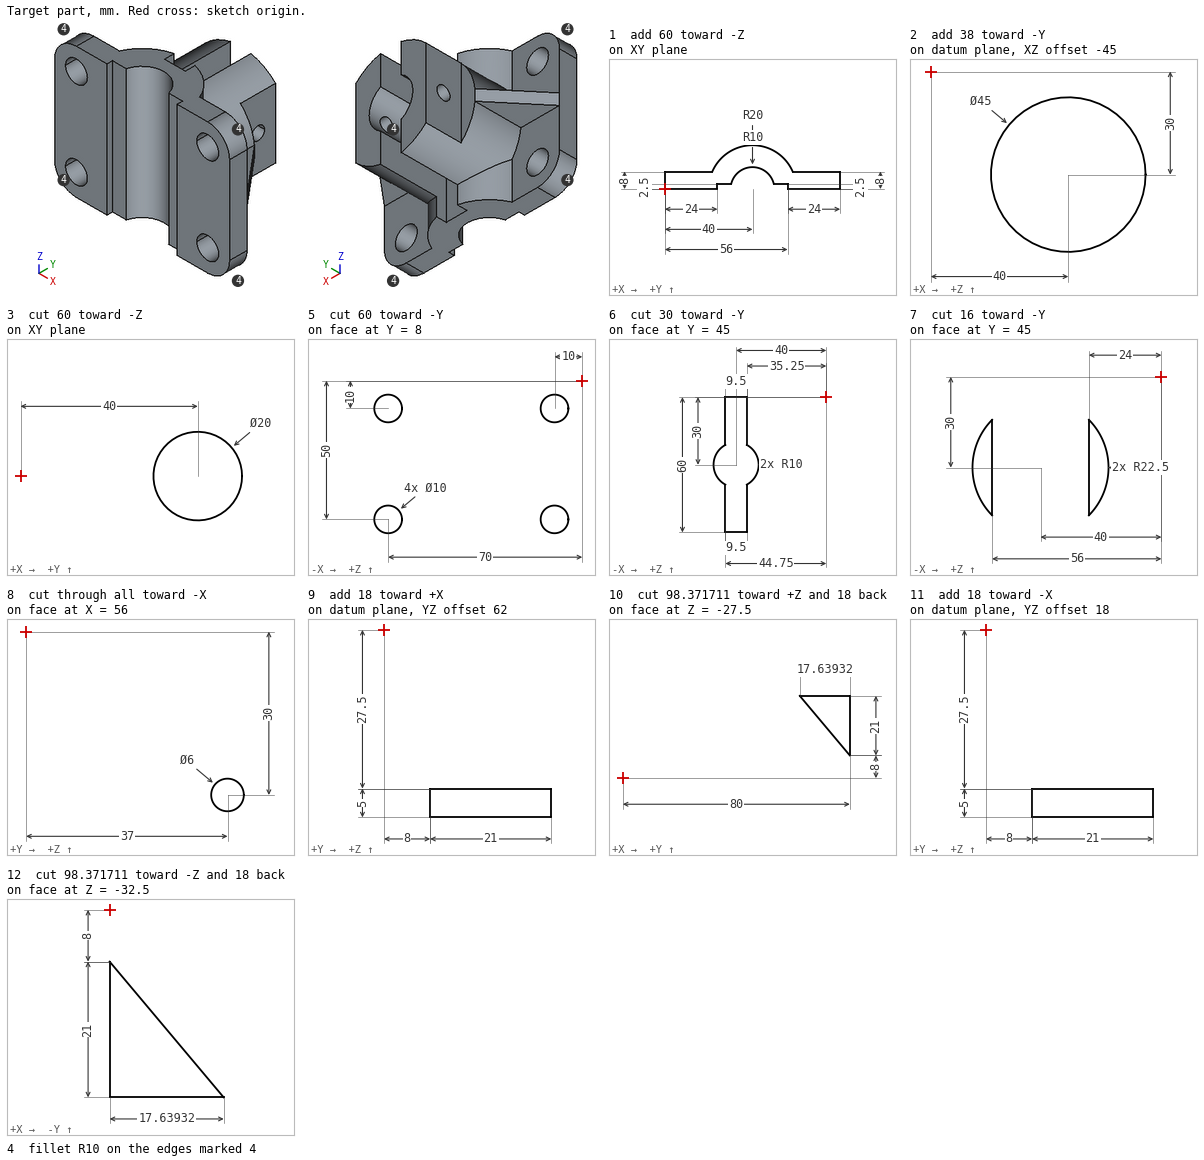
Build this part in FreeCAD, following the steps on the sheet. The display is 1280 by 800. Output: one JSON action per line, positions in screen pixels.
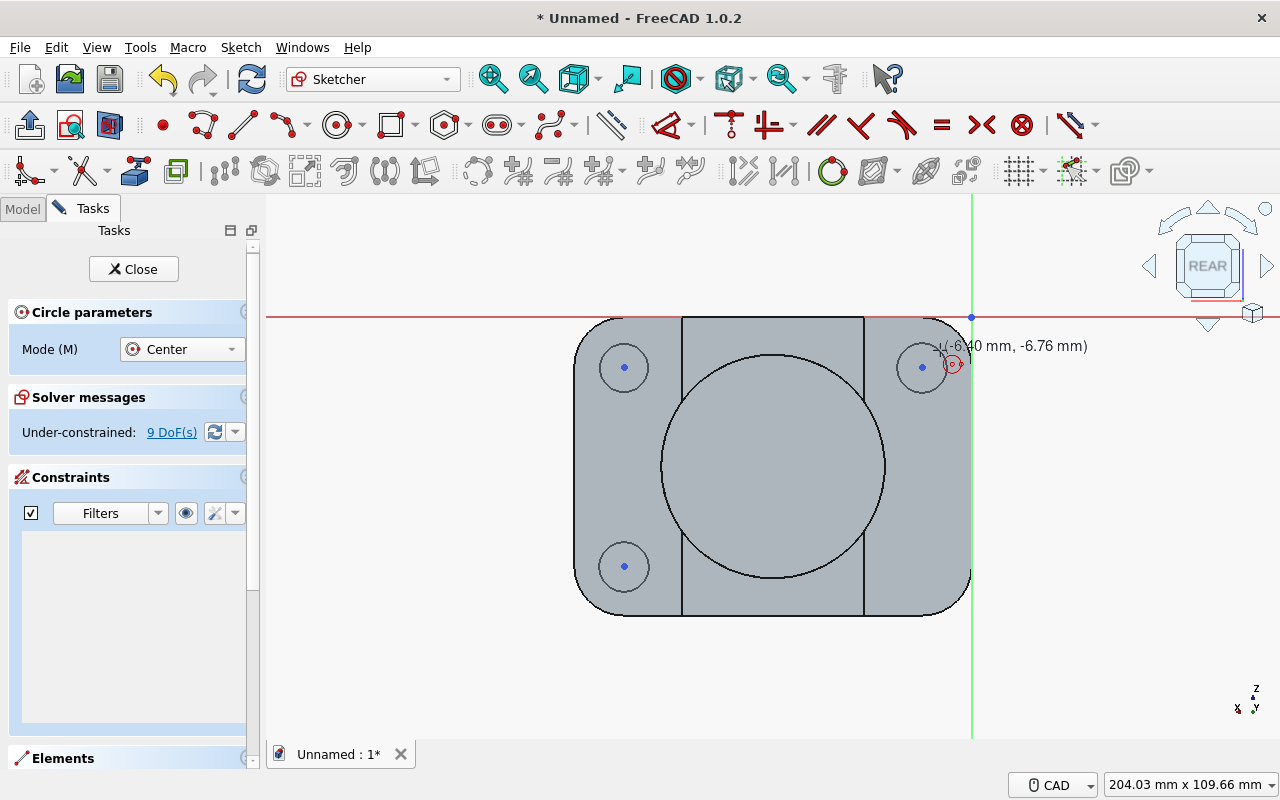
{"action": "left_click", "coordinate": [922, 566]}
{"action": "left_click", "coordinate": [940, 548]}
{"action": "key", "text": "Escape"}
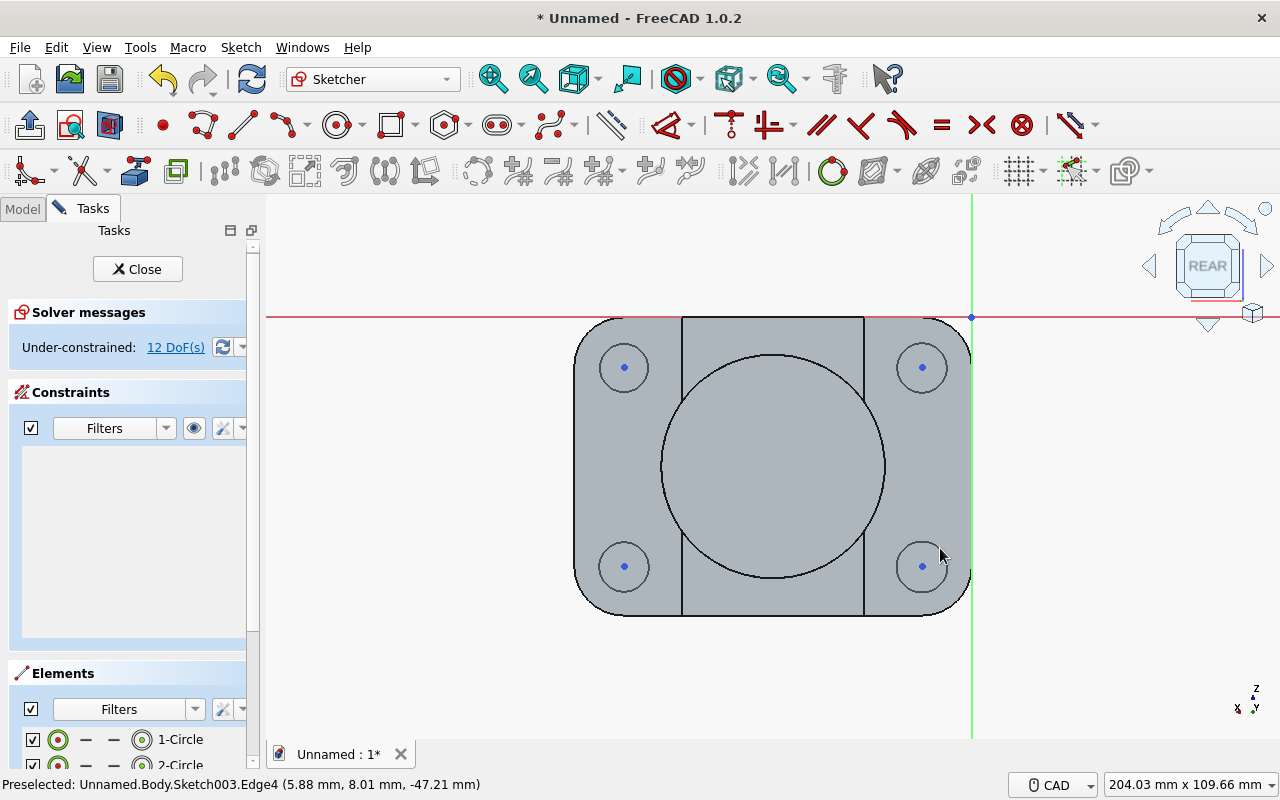
{"action": "left_click", "coordinate": [641, 549]}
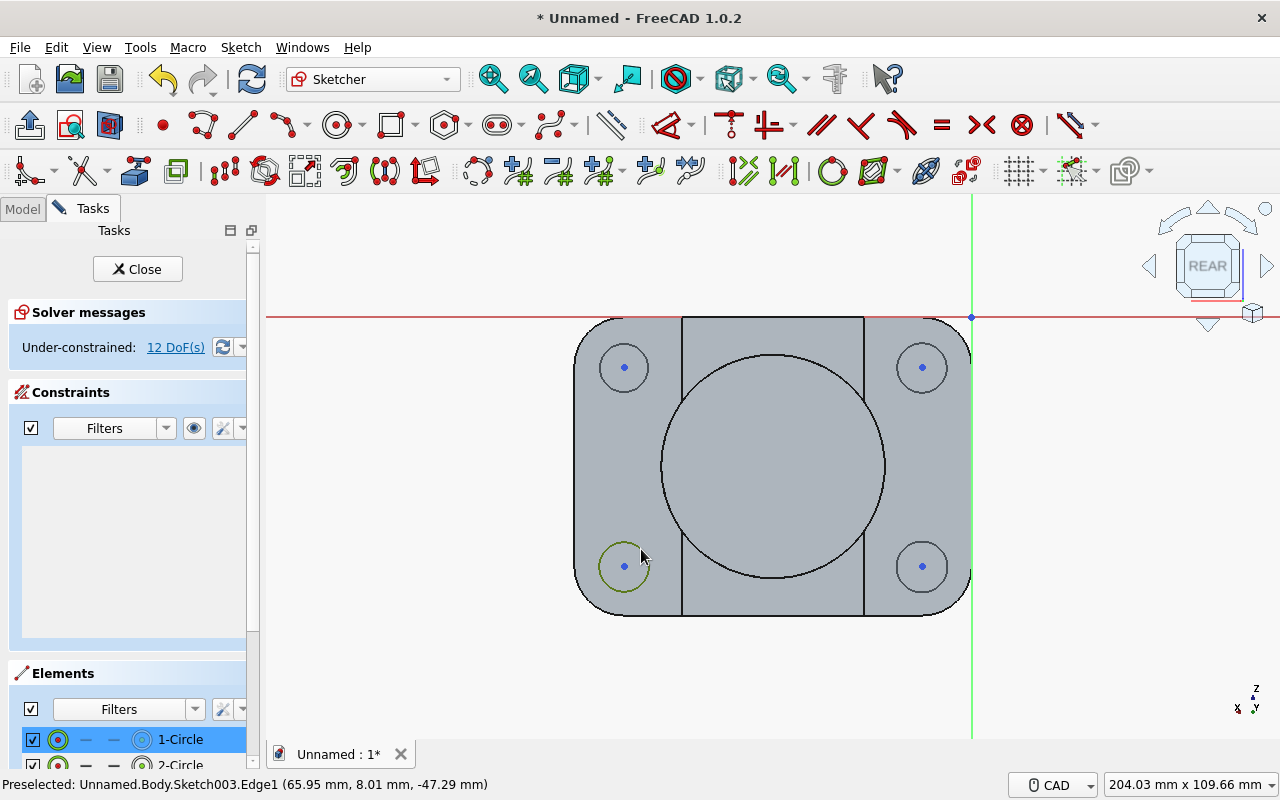
{"action": "left_click", "coordinate": [641, 351]}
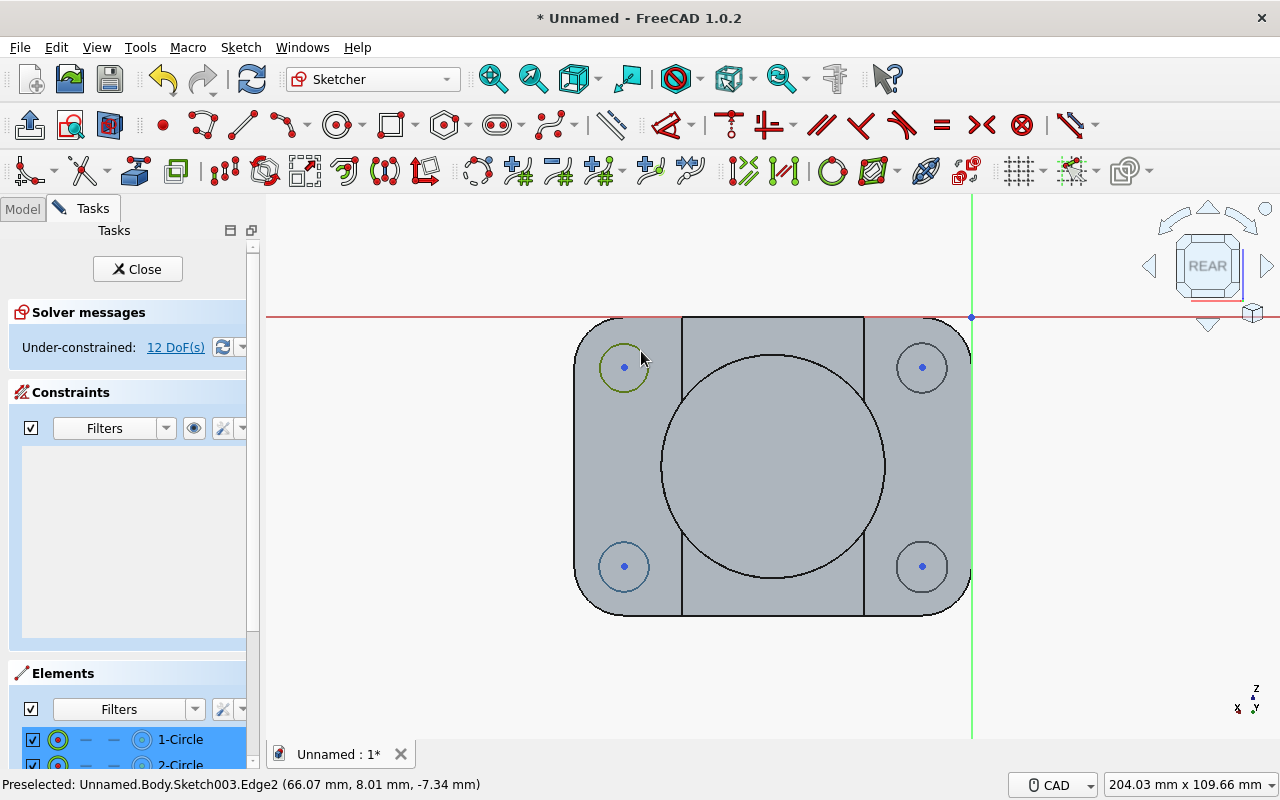
{"action": "left_click", "coordinate": [939, 350]}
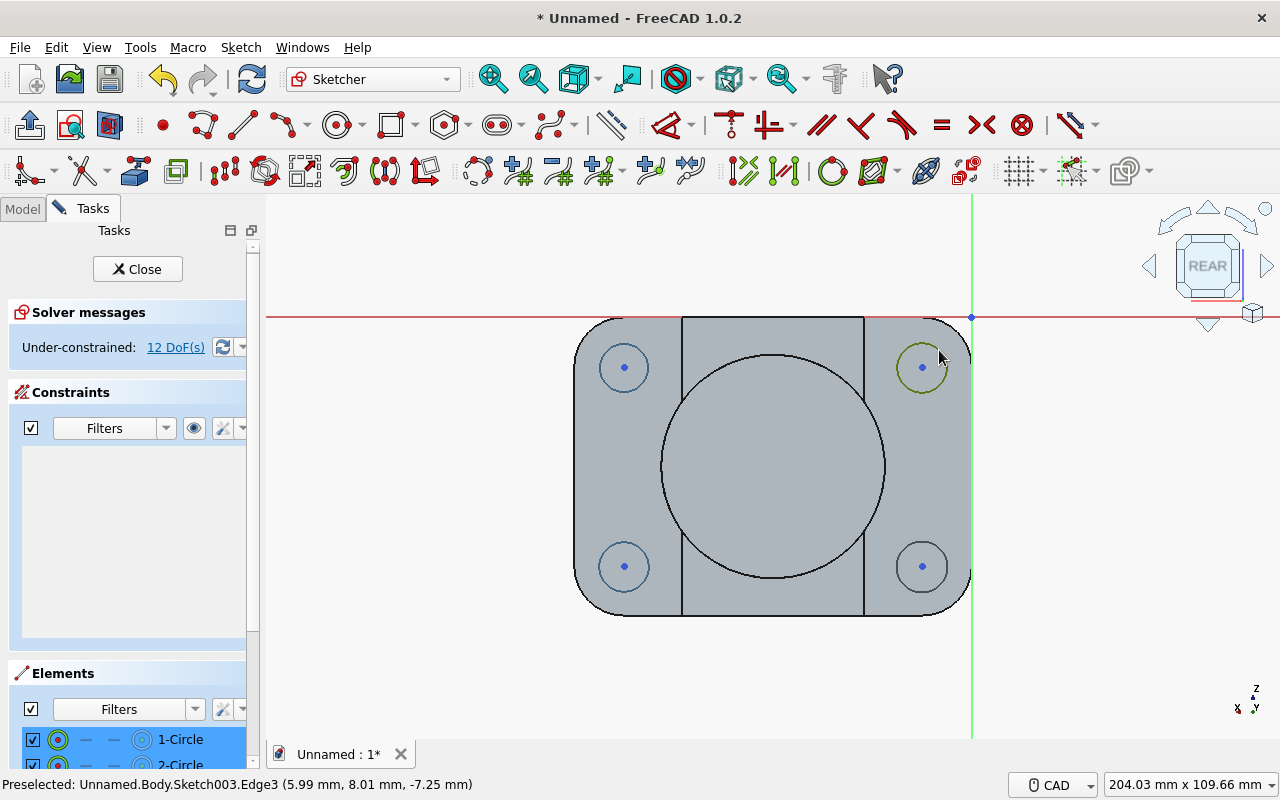
{"action": "left_click", "coordinate": [940, 549]}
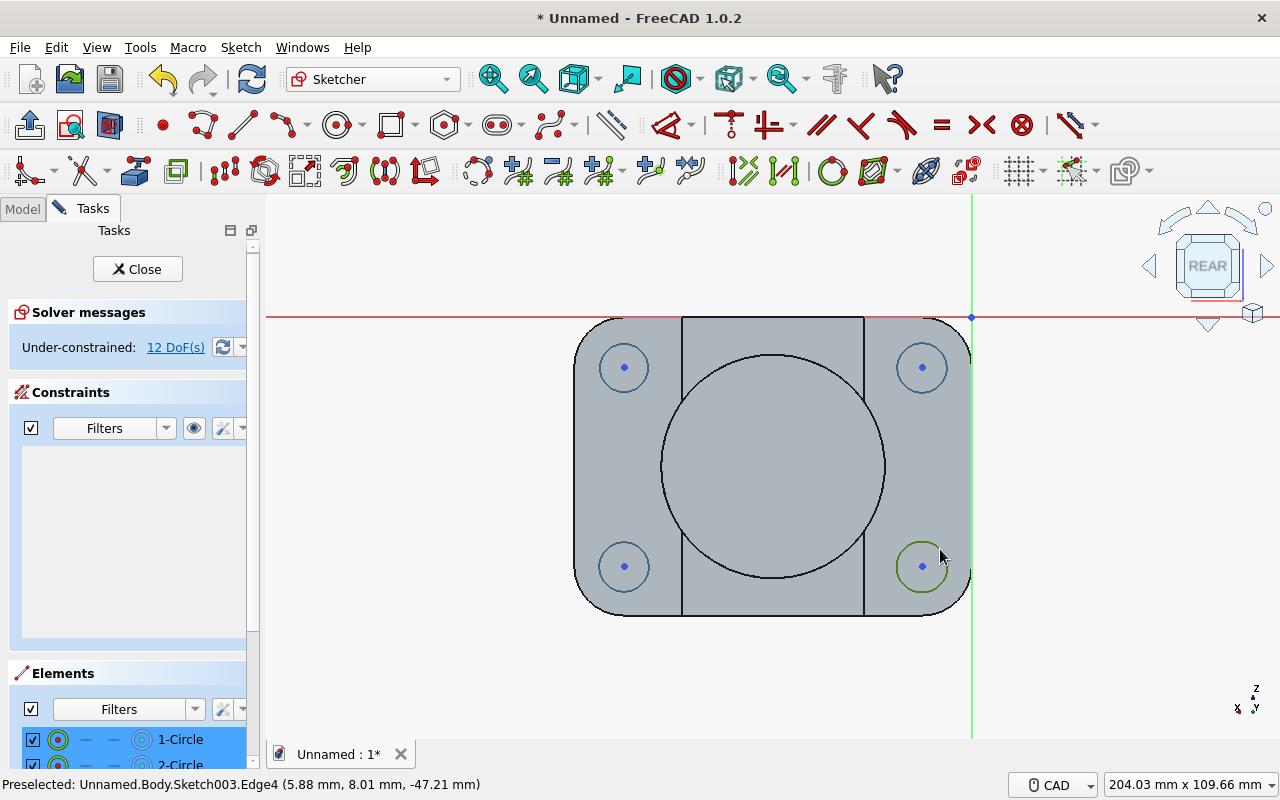
{"action": "left_click", "coordinate": [942, 126]}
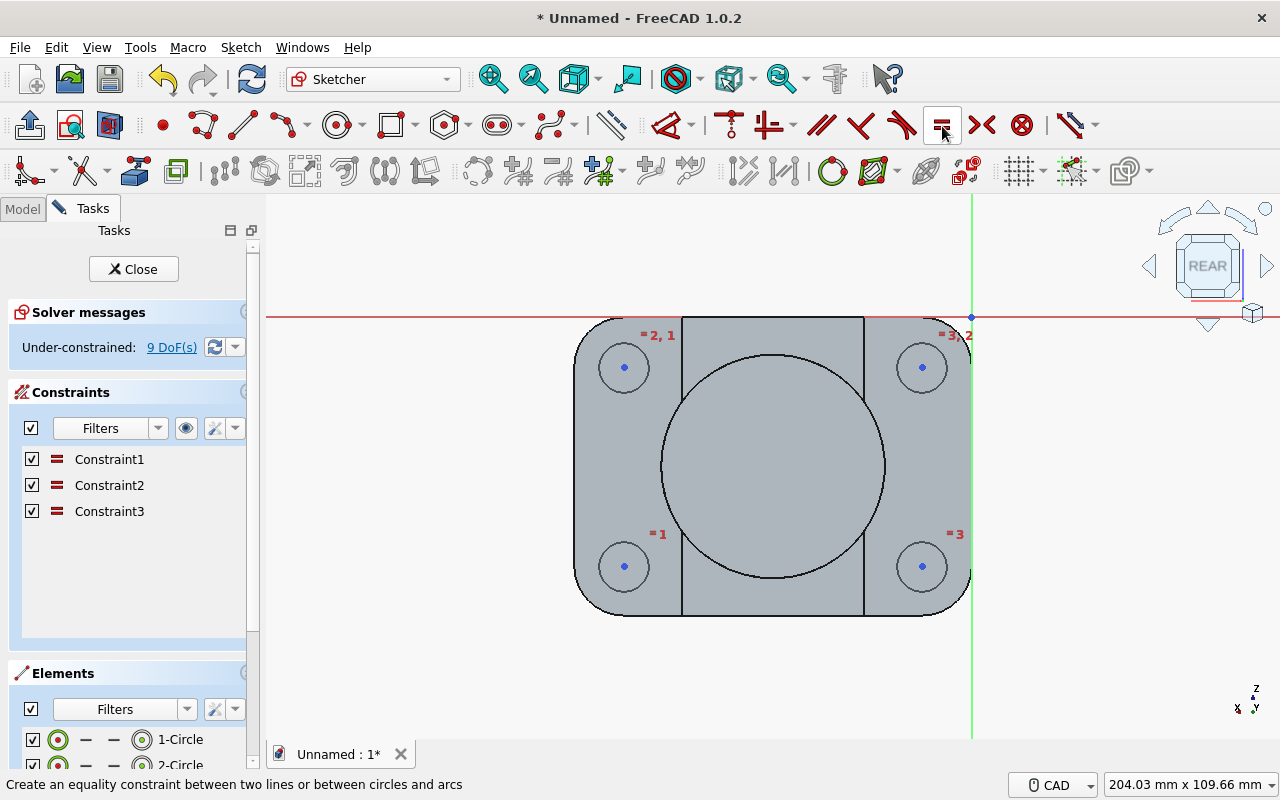
{"action": "left_click", "coordinate": [624, 567]}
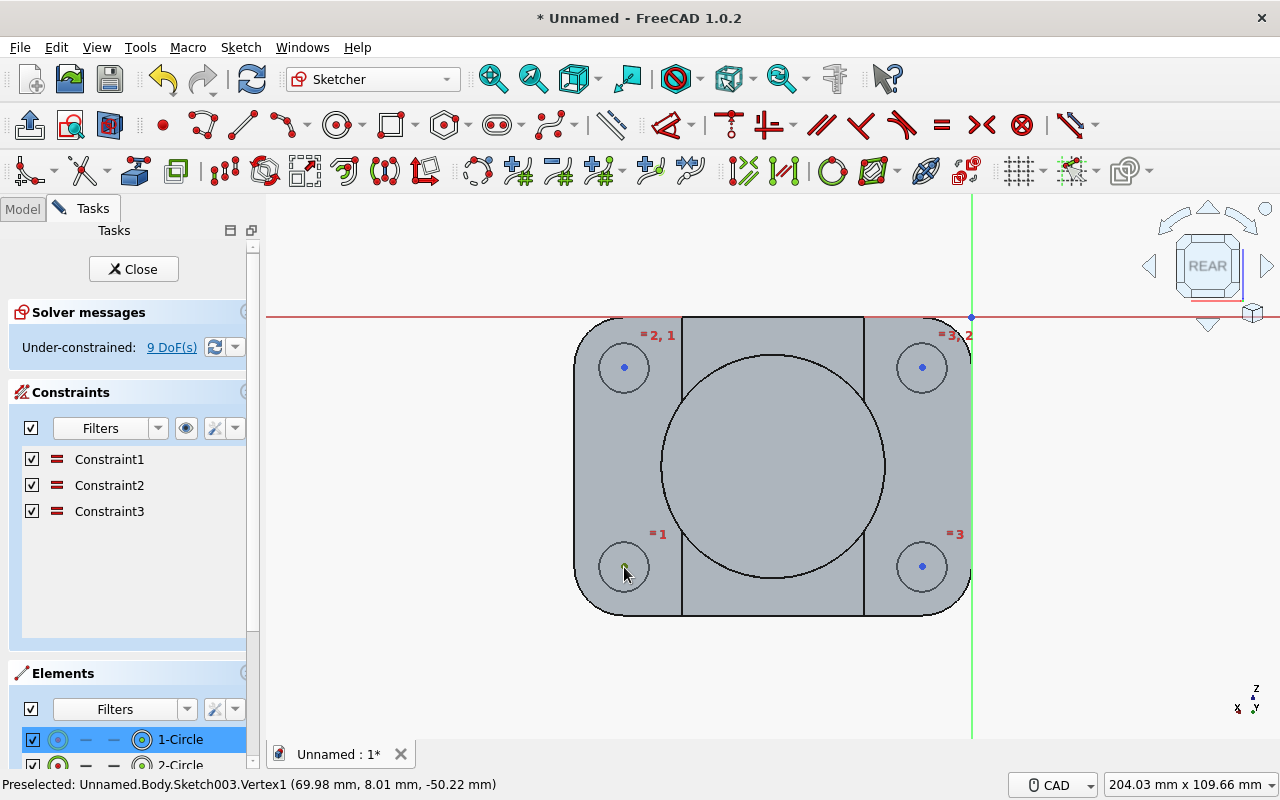
{"action": "left_click", "coordinate": [624, 368]}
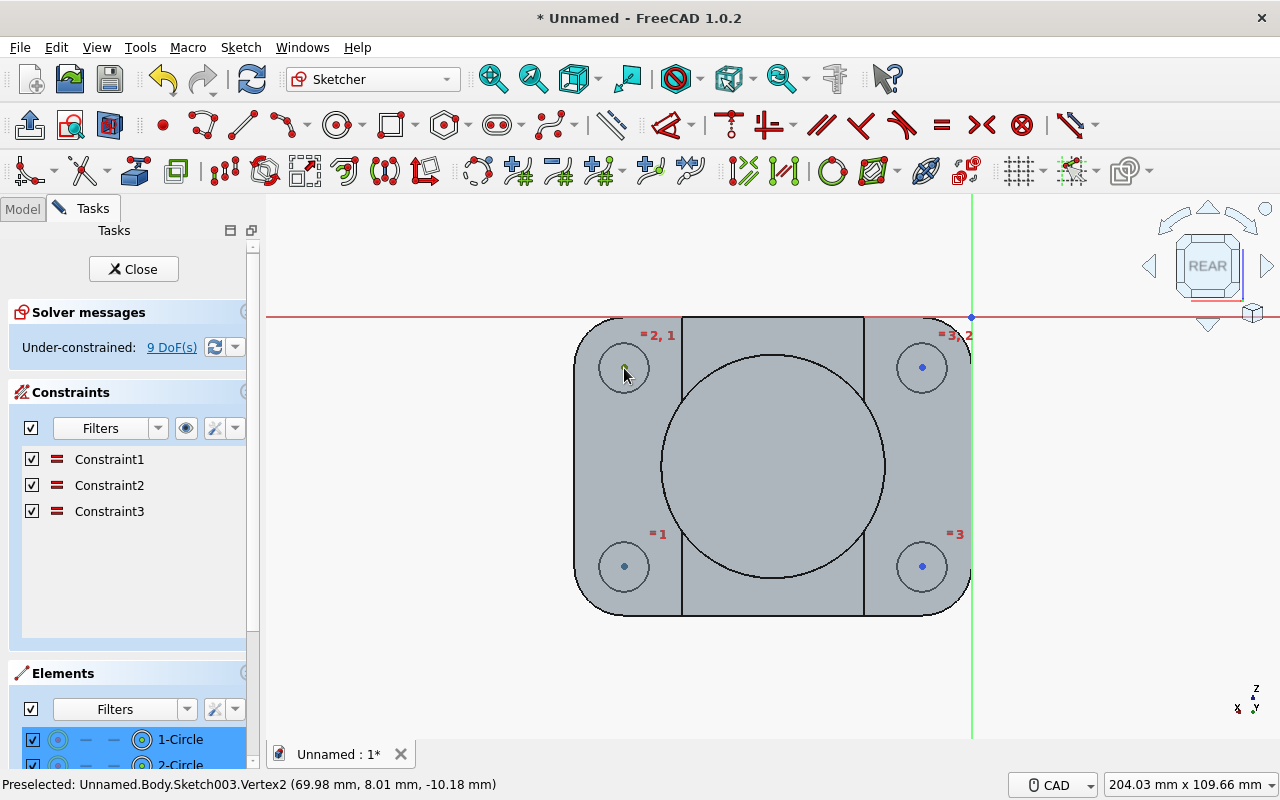
{"action": "left_click", "coordinate": [796, 126]}